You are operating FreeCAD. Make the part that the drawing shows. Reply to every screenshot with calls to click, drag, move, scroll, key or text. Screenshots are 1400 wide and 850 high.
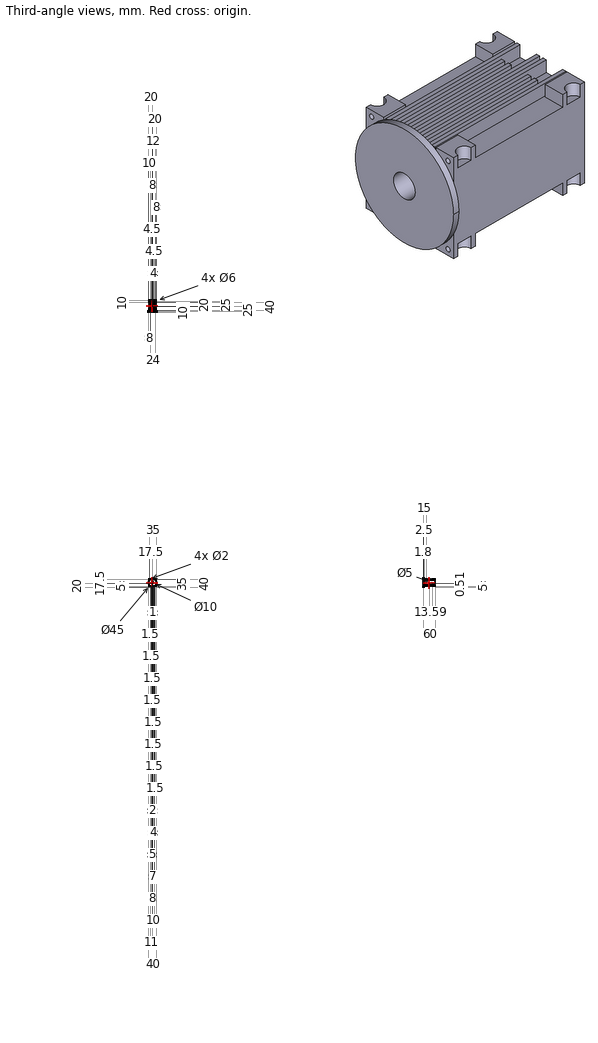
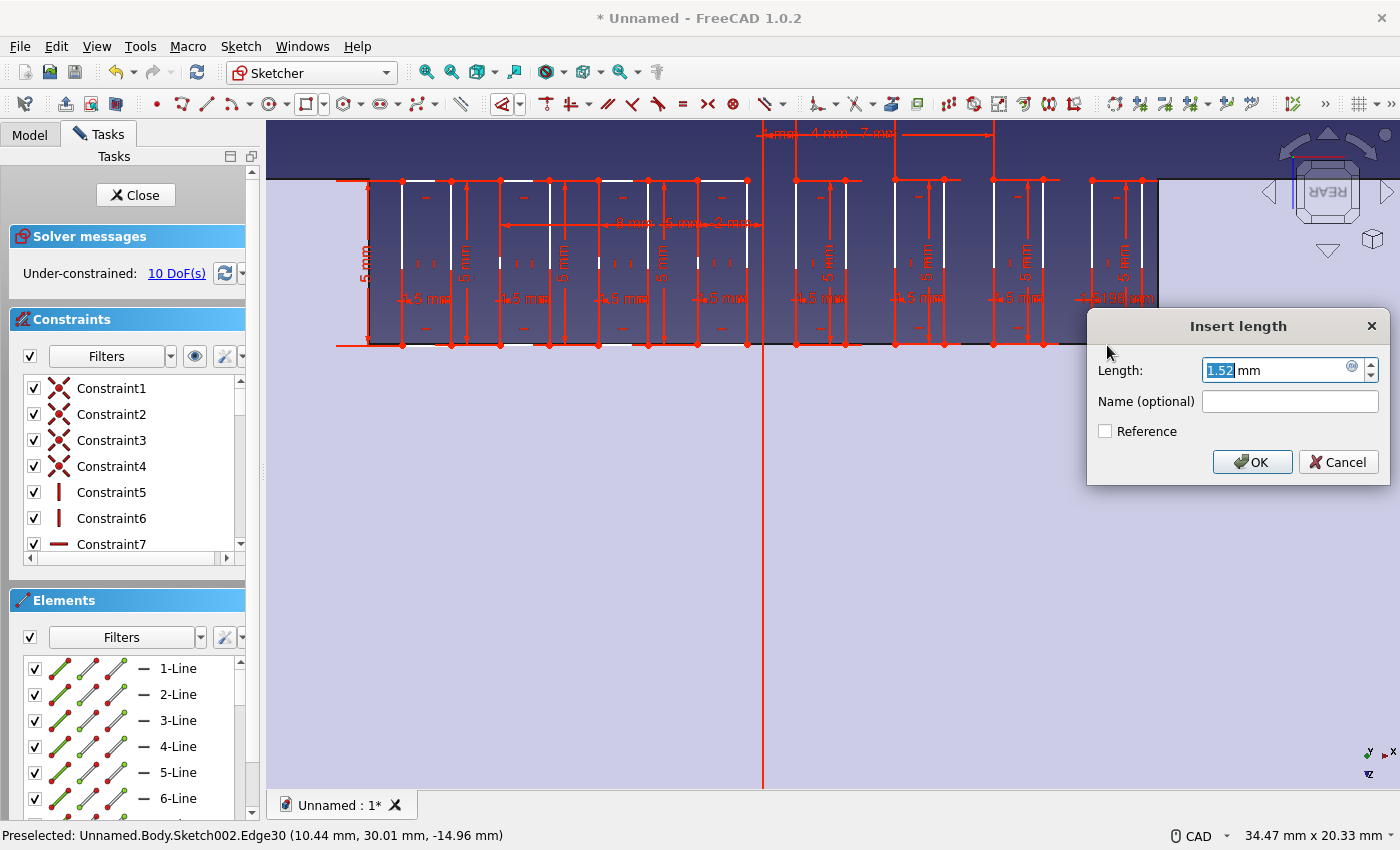
text(1.5)
key(Return)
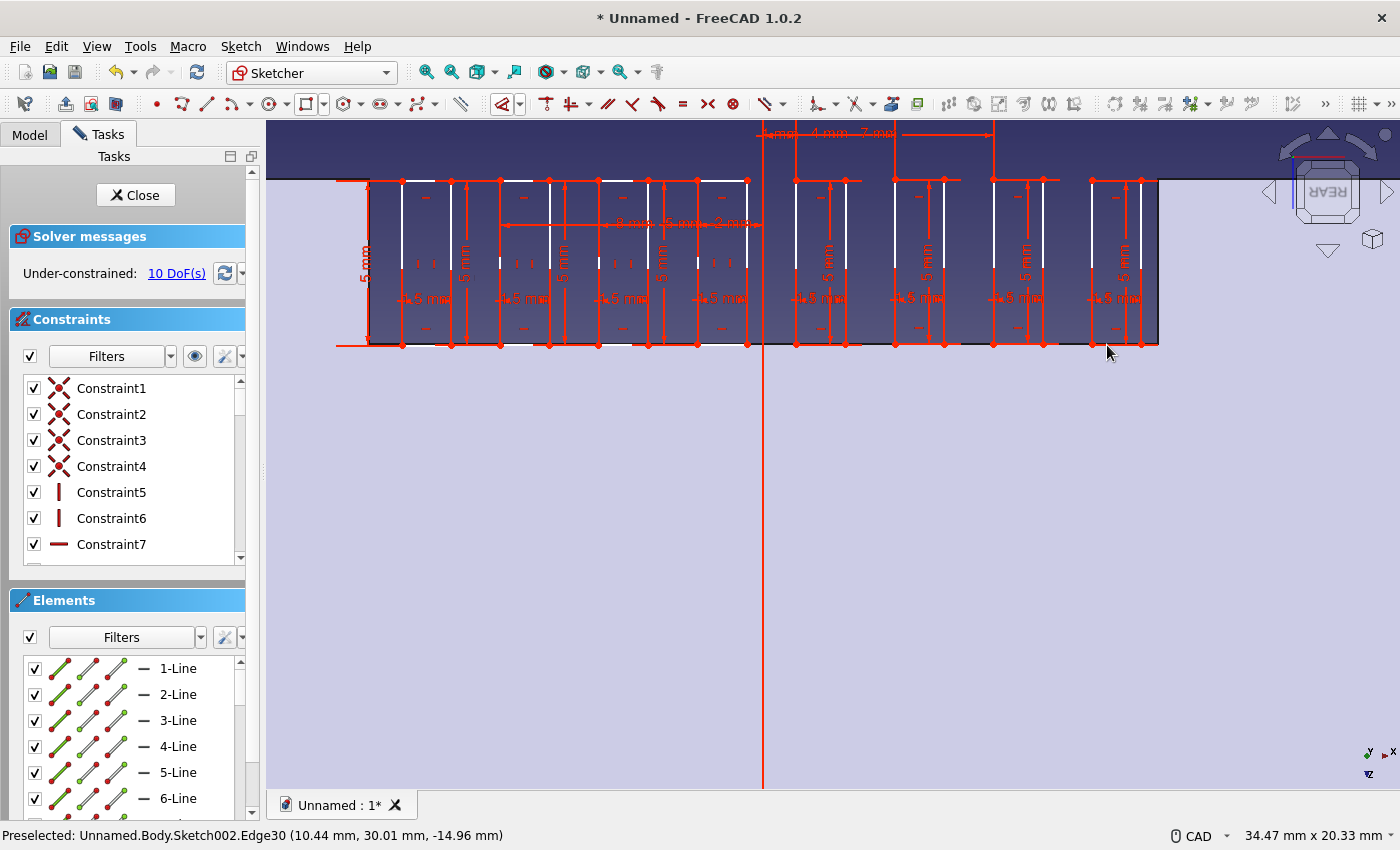
click(402, 181)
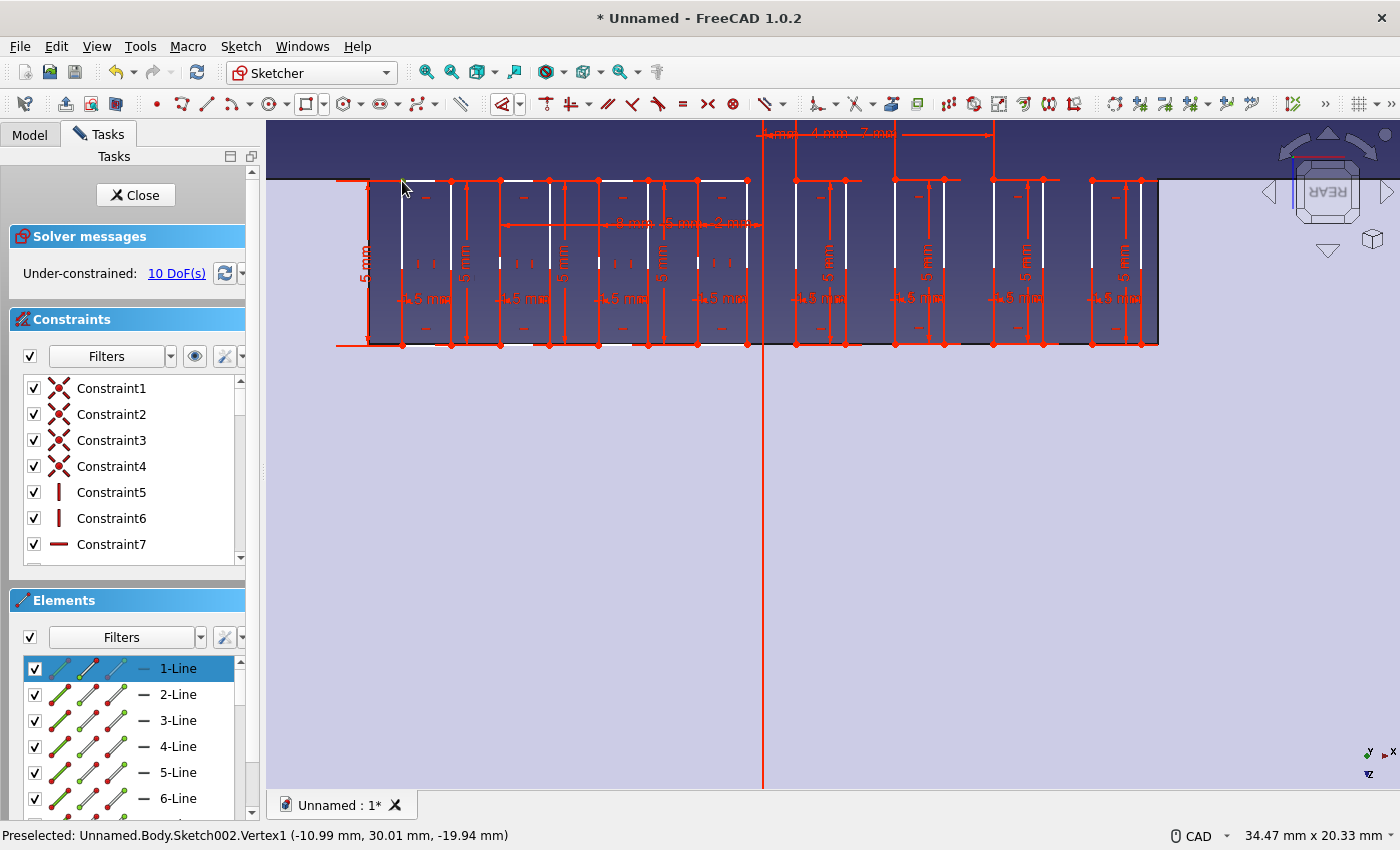
key(l)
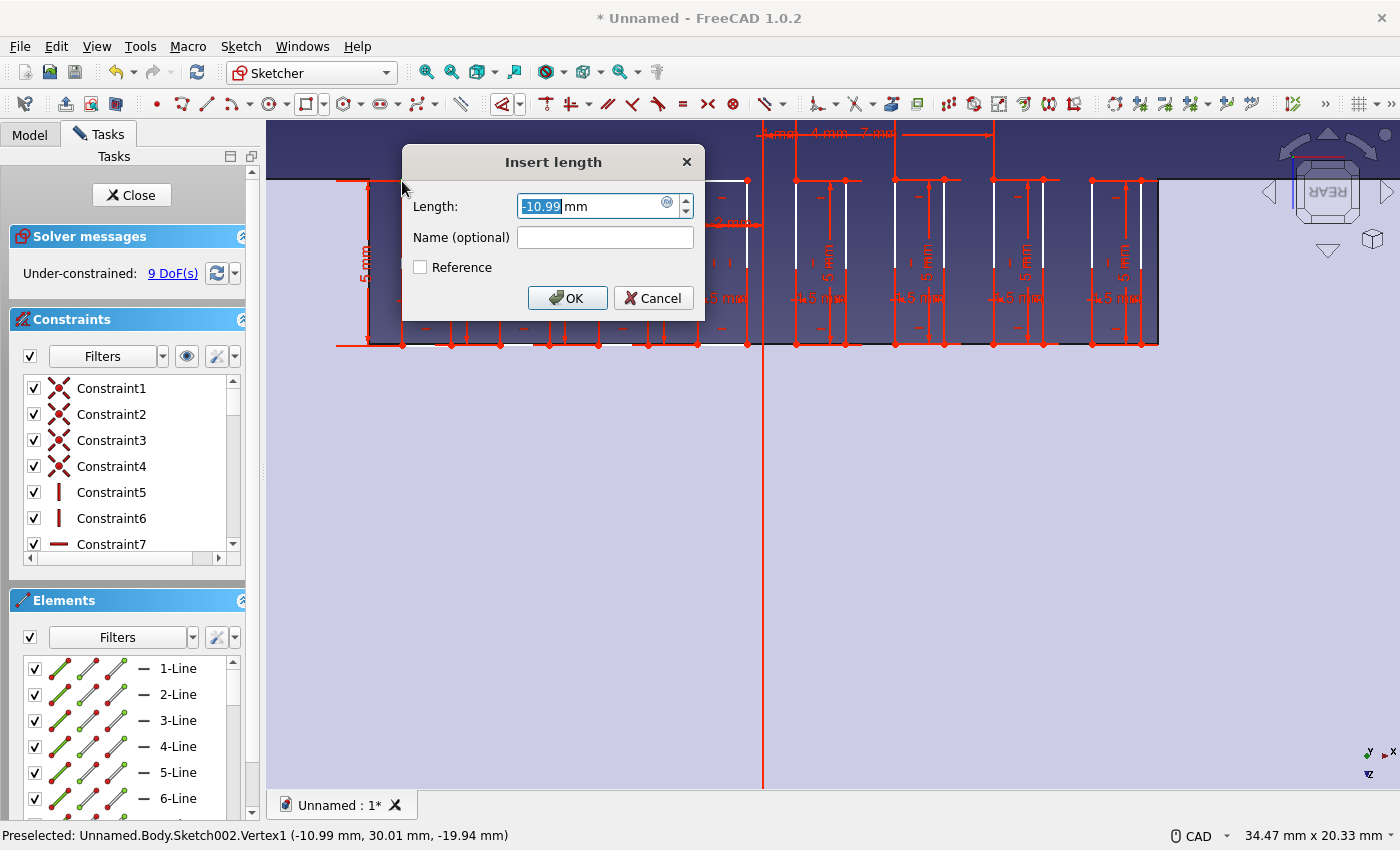
text(-11)
key(Return)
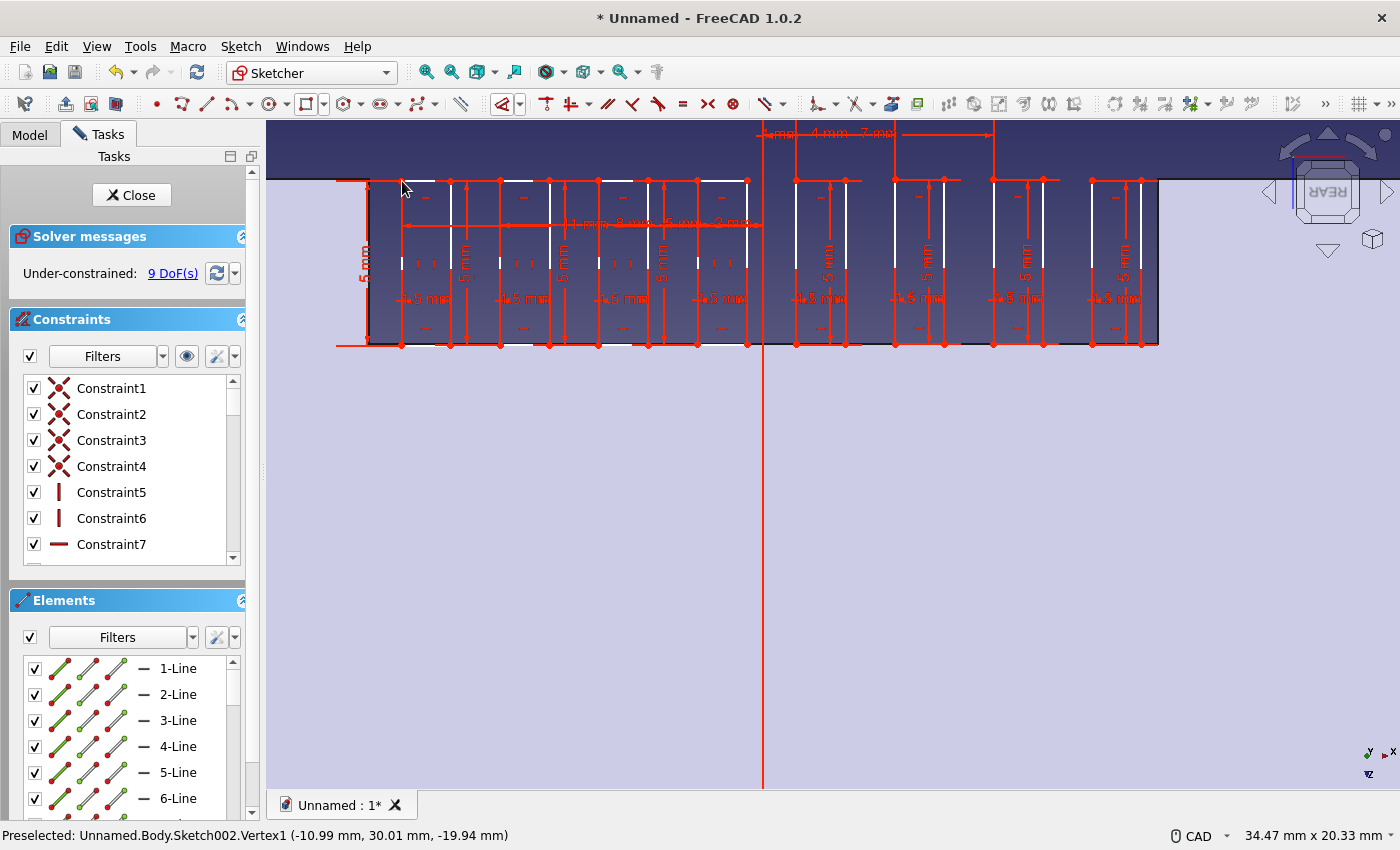
click(402, 181)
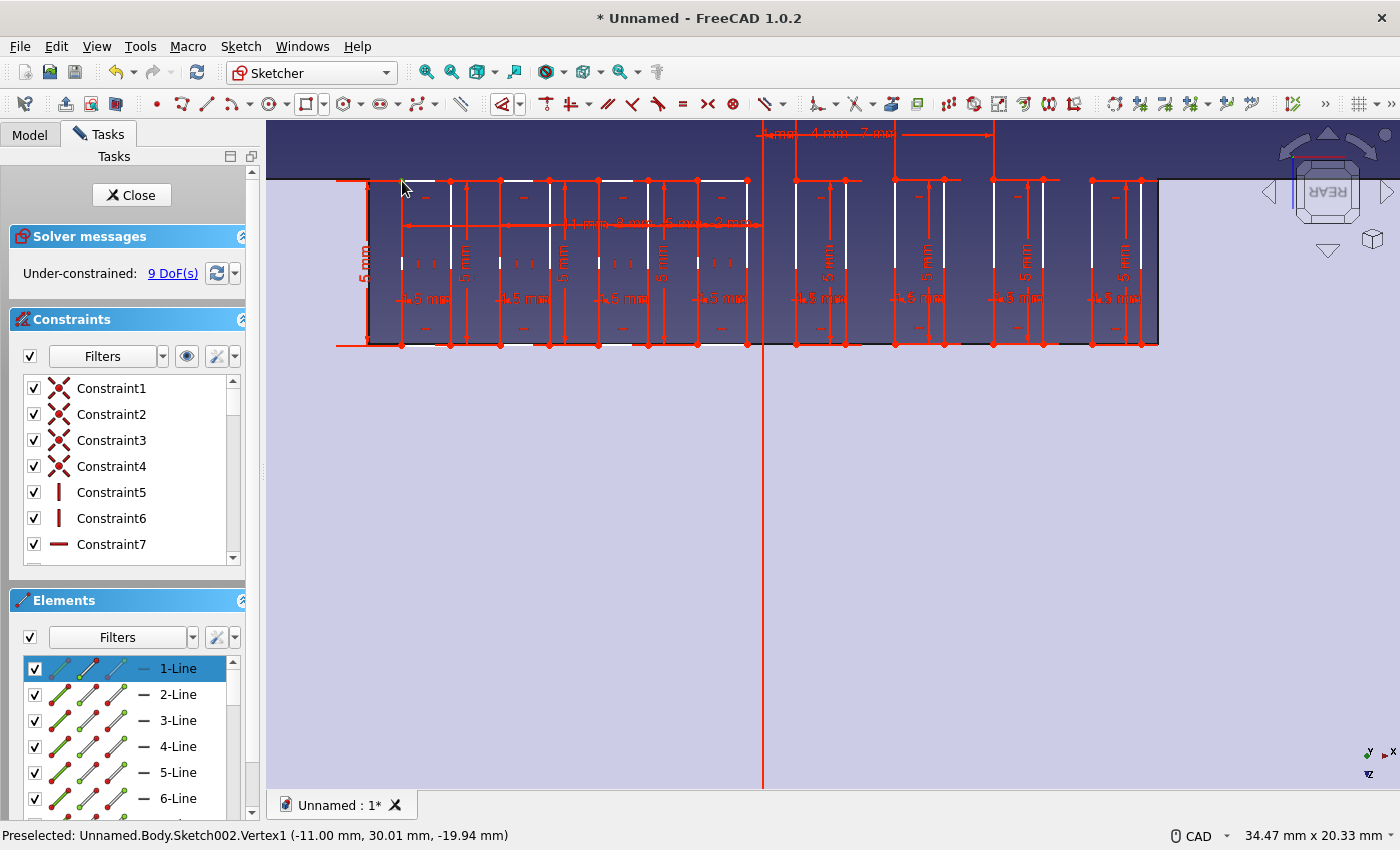
click(520, 104)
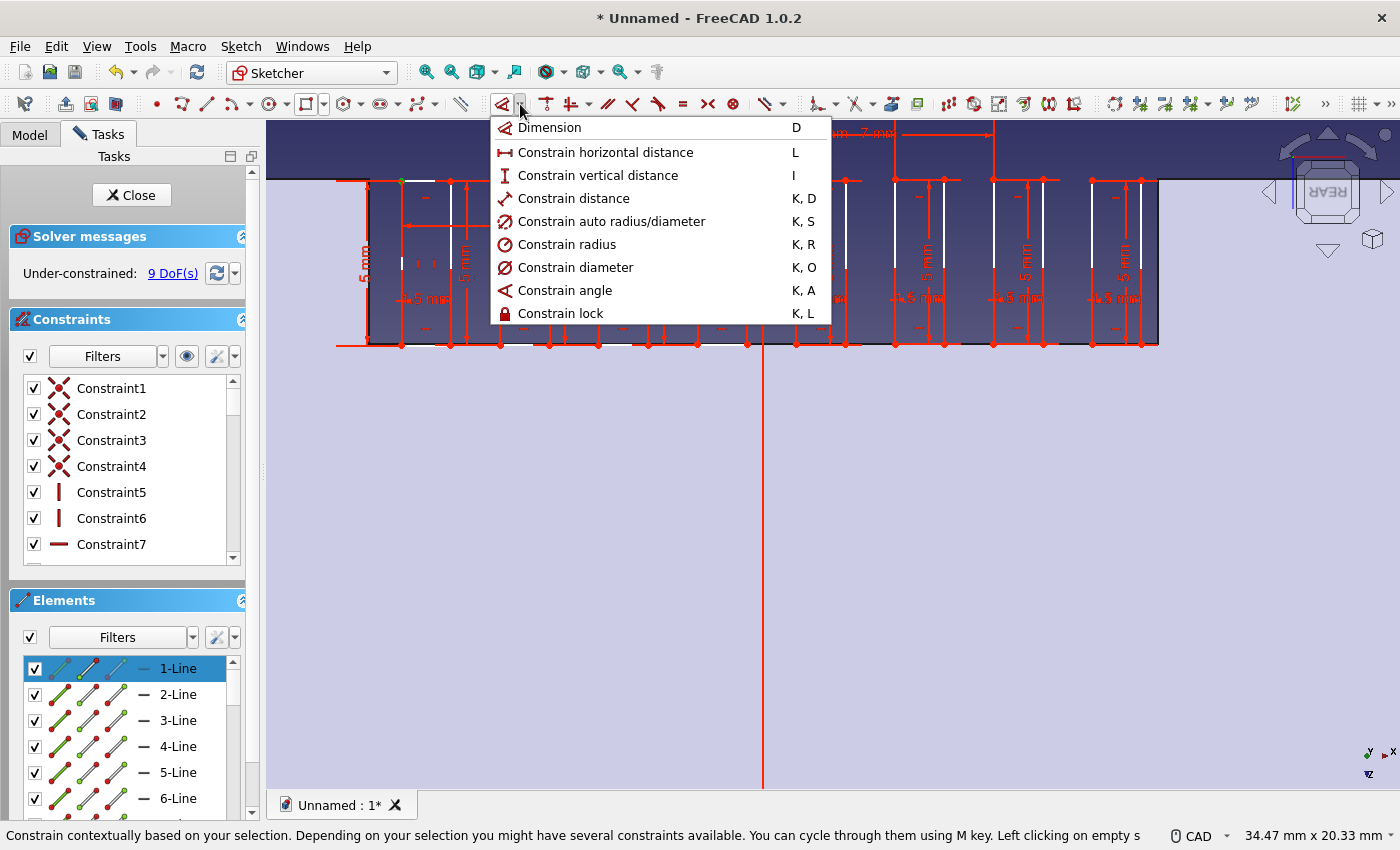
click(661, 176)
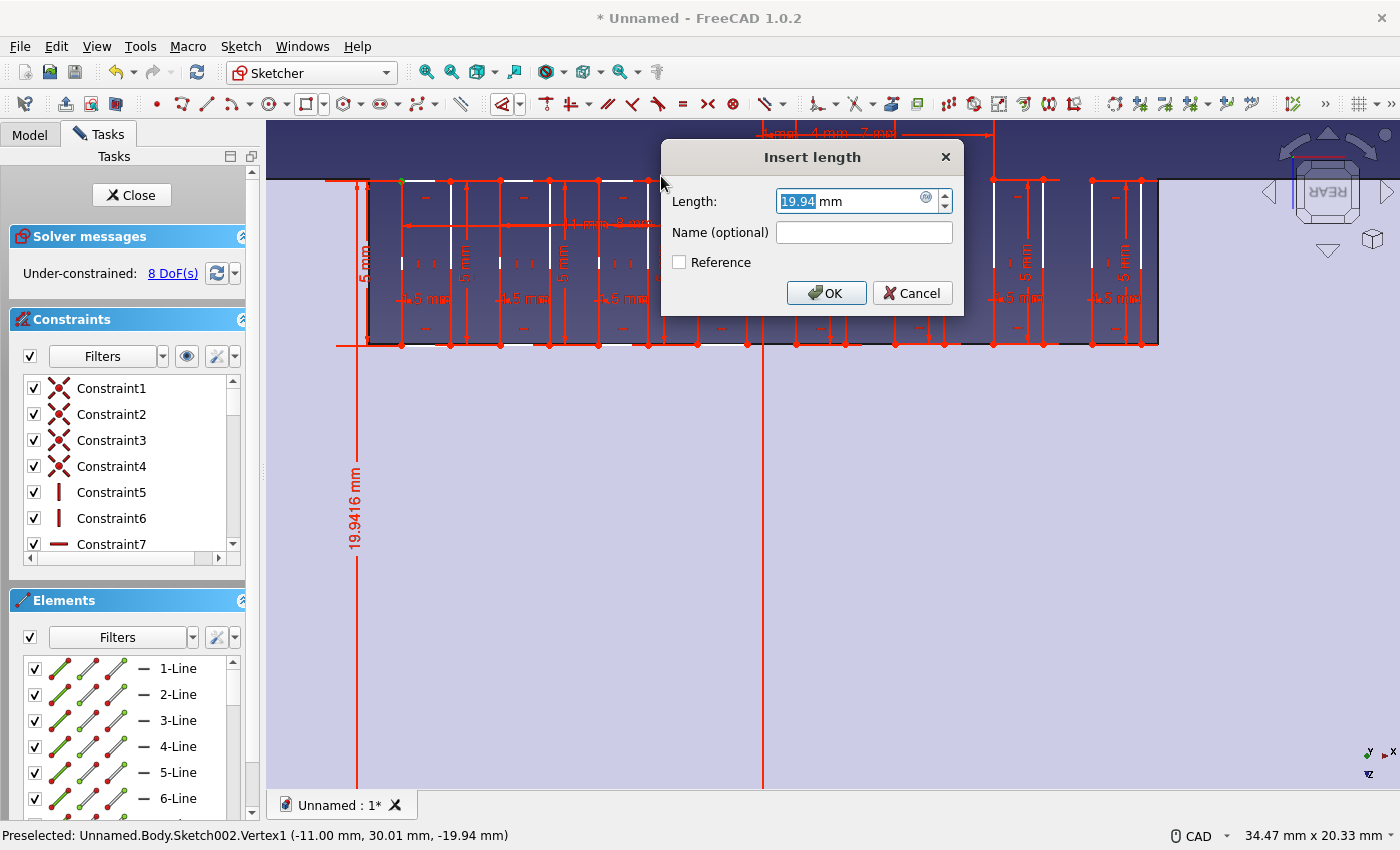
text(20)
key(Return)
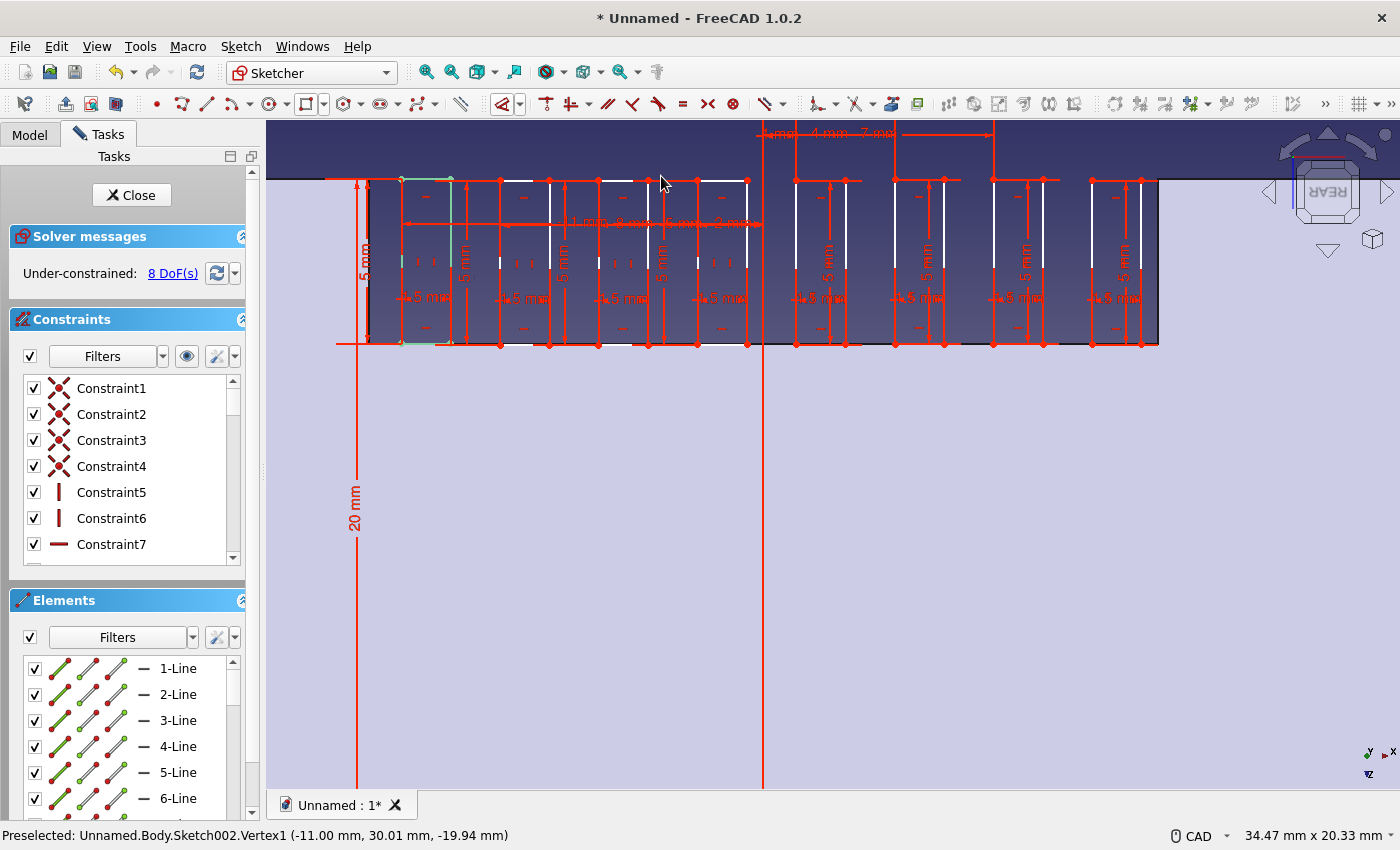
click(500, 181)